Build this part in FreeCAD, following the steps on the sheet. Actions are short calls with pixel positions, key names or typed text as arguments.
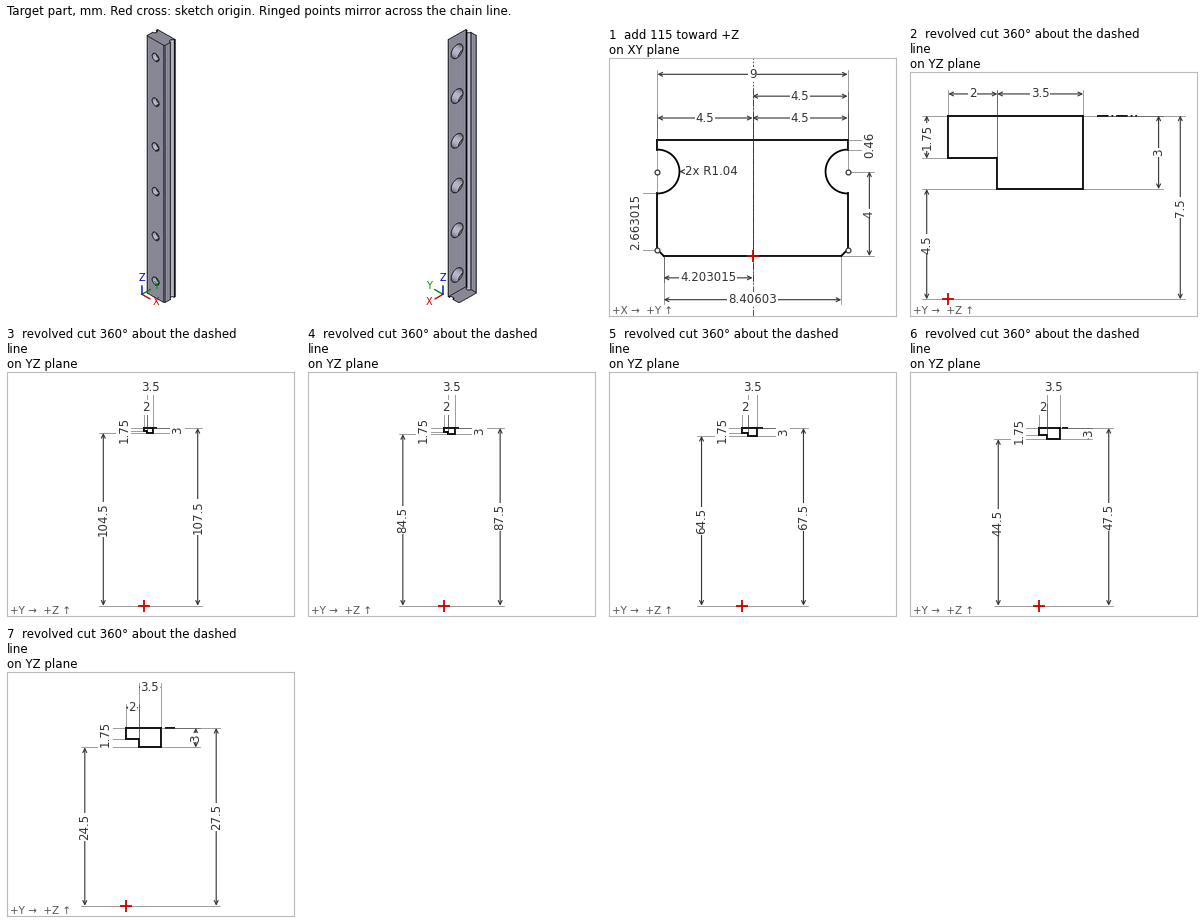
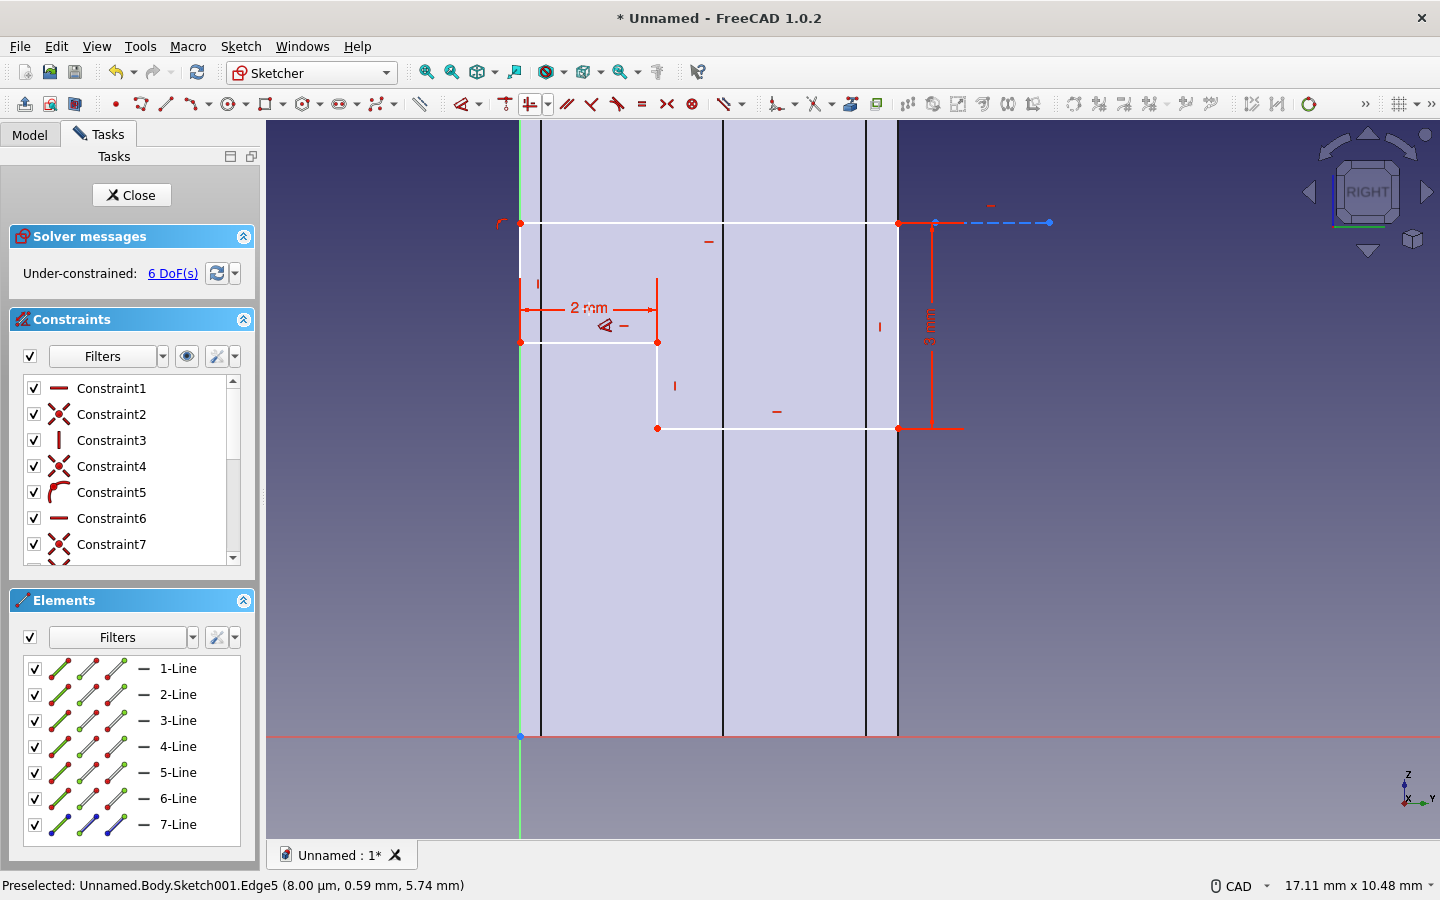
click(730, 429)
click(778, 395)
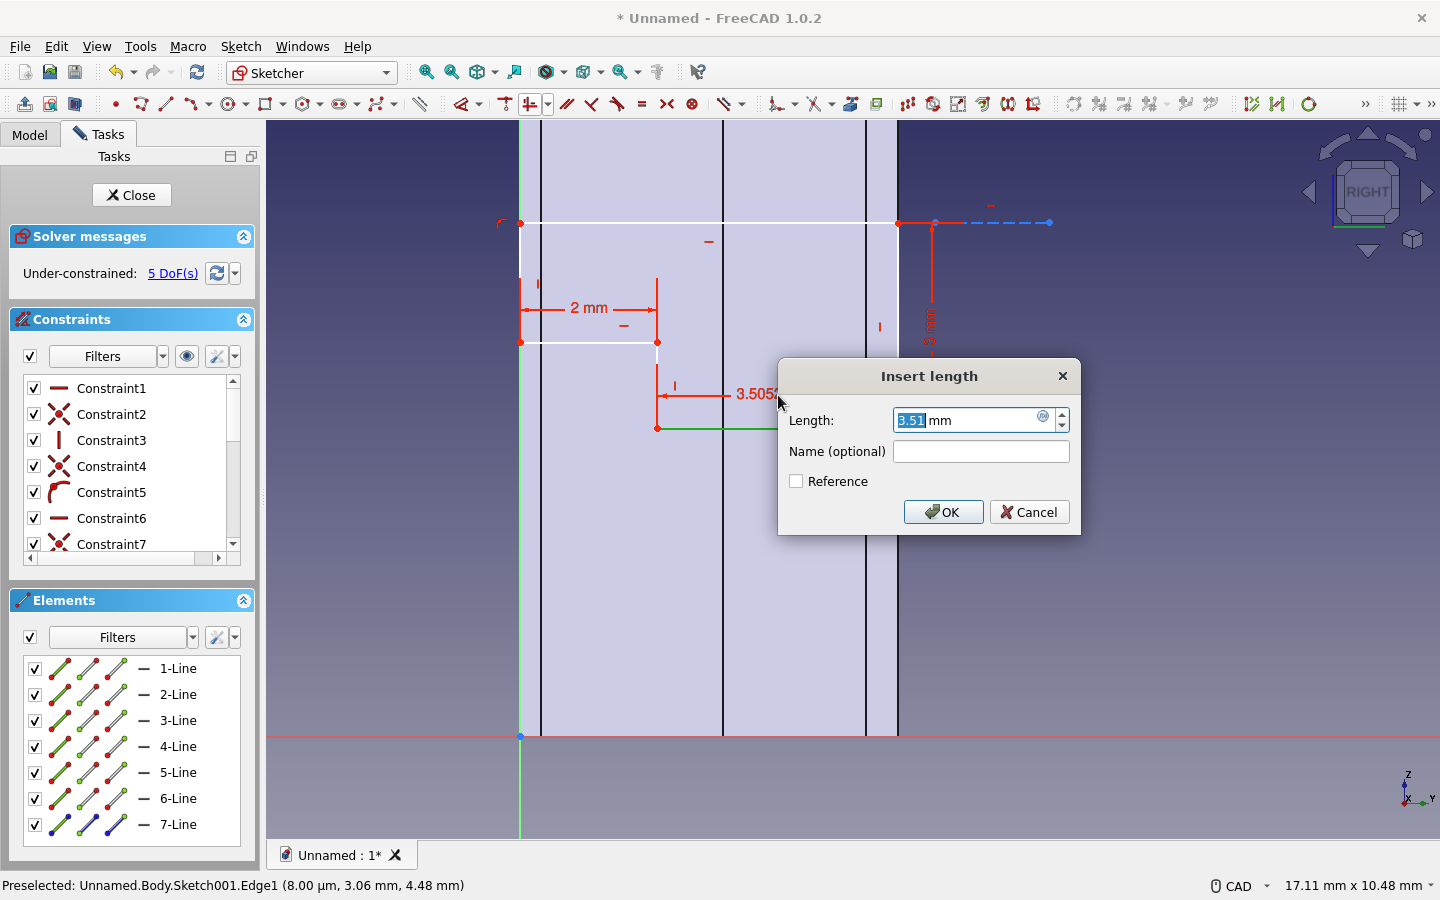
text(3.5)
key(Return)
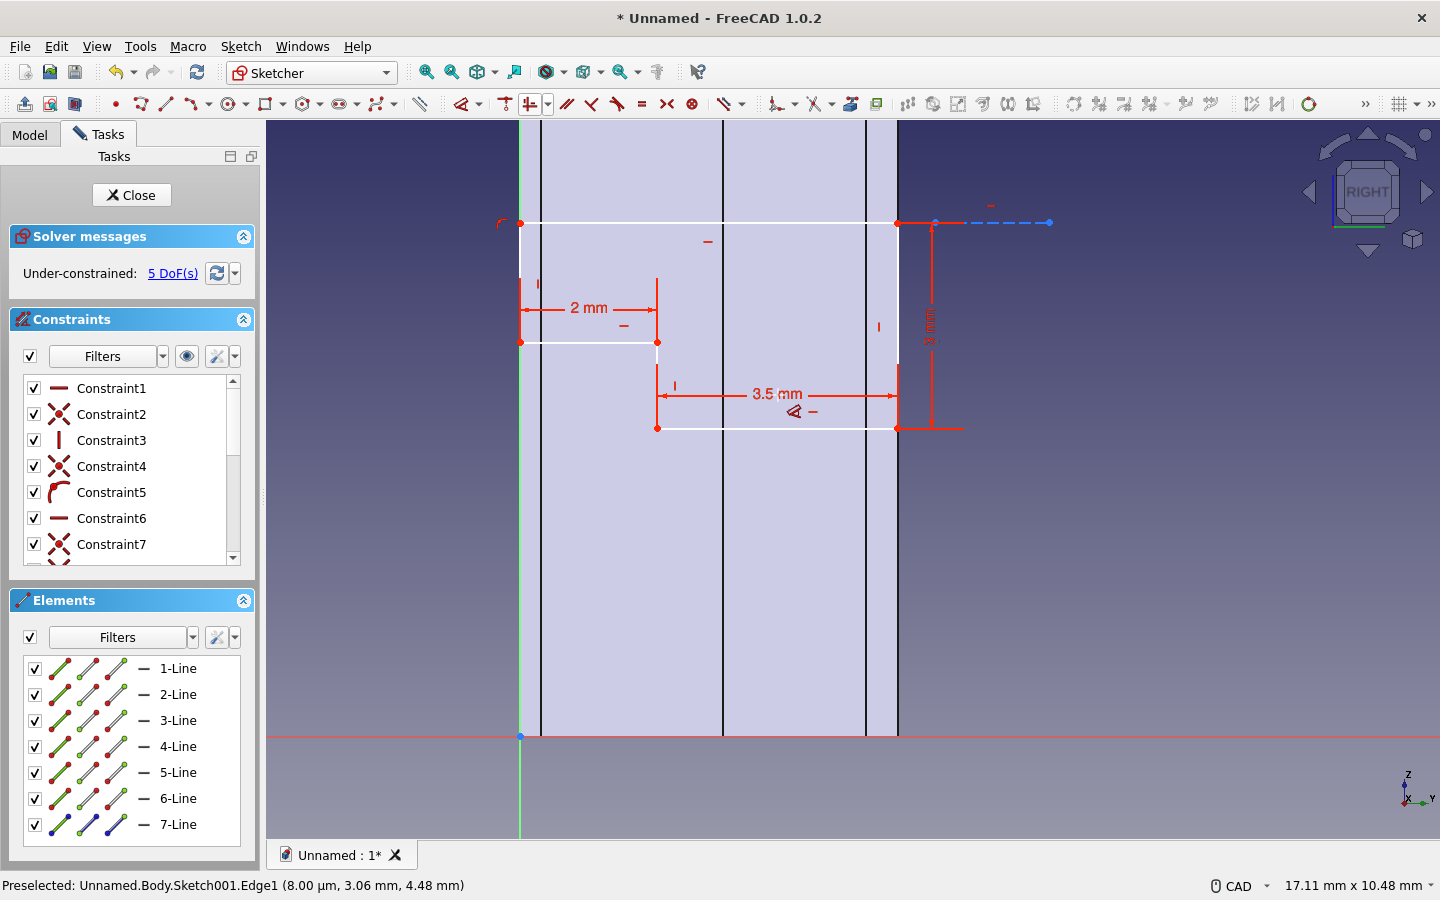
click(520, 259)
click(486, 283)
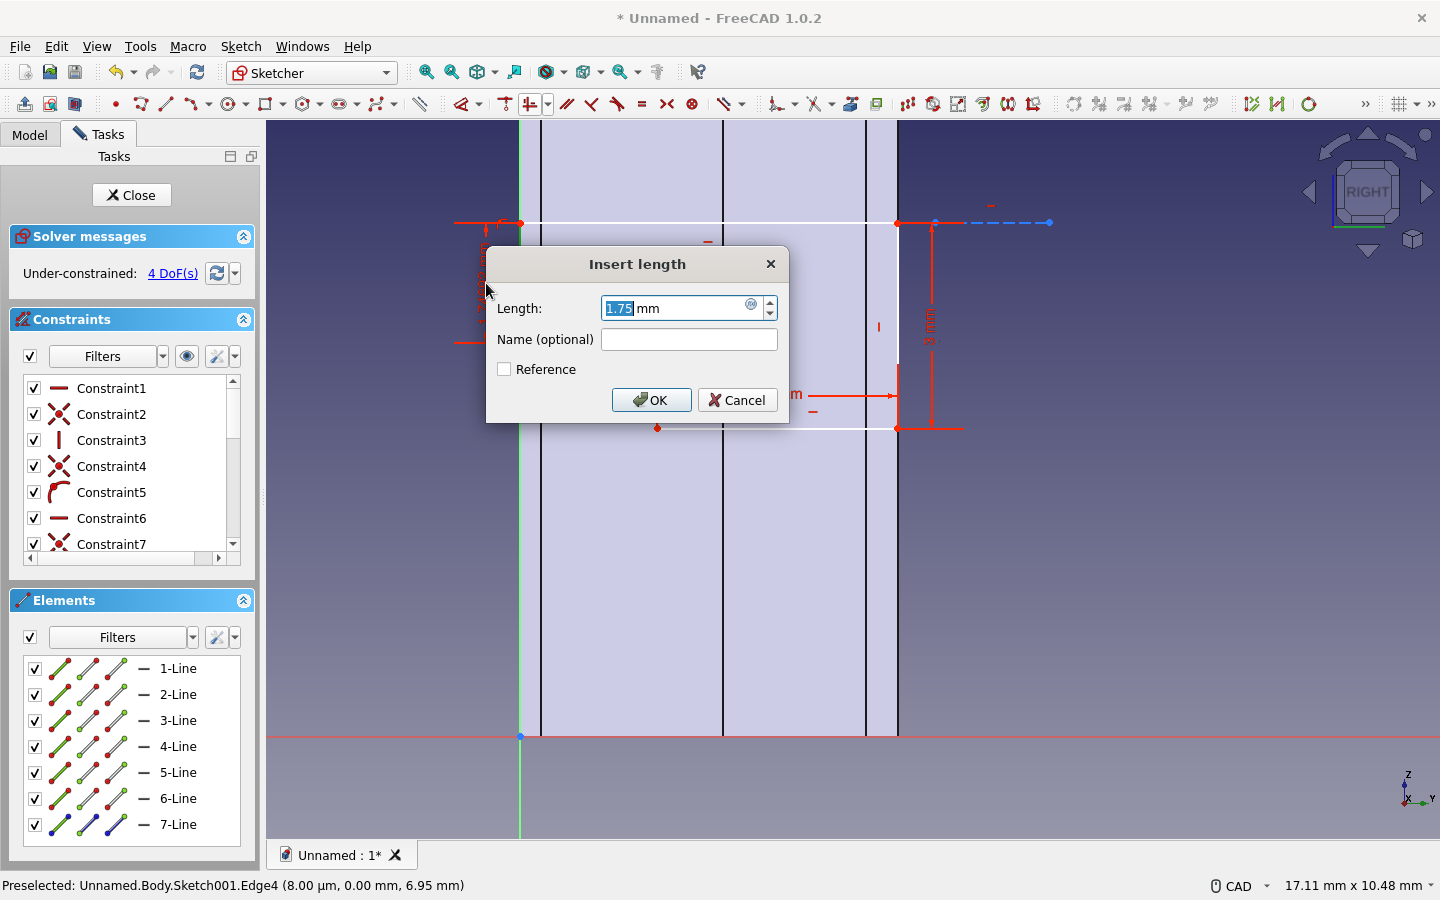
text(1.75)
key(Return)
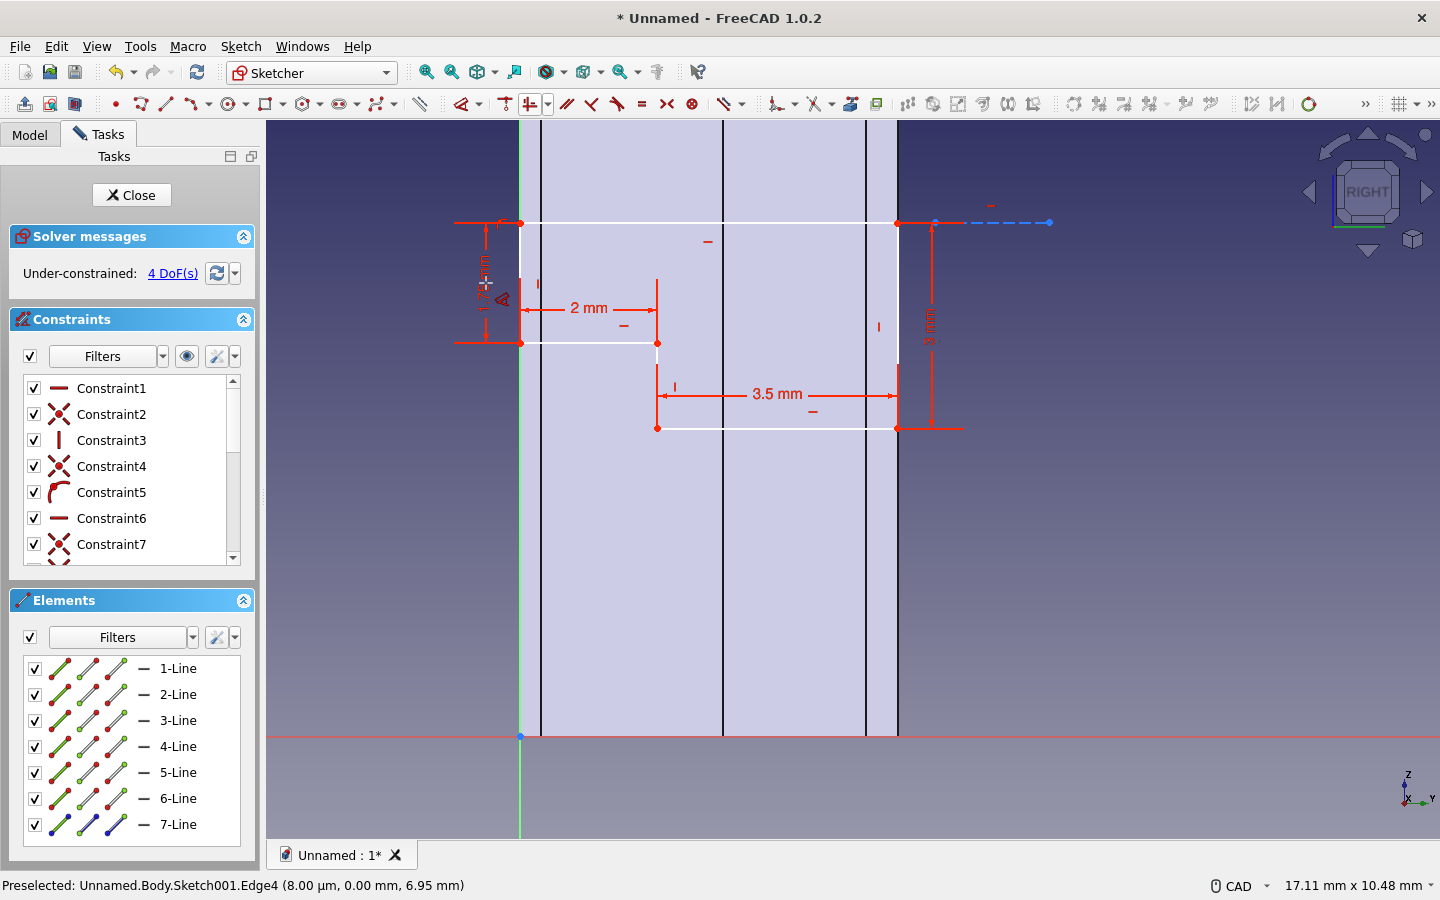
click(657, 429)
click(486, 583)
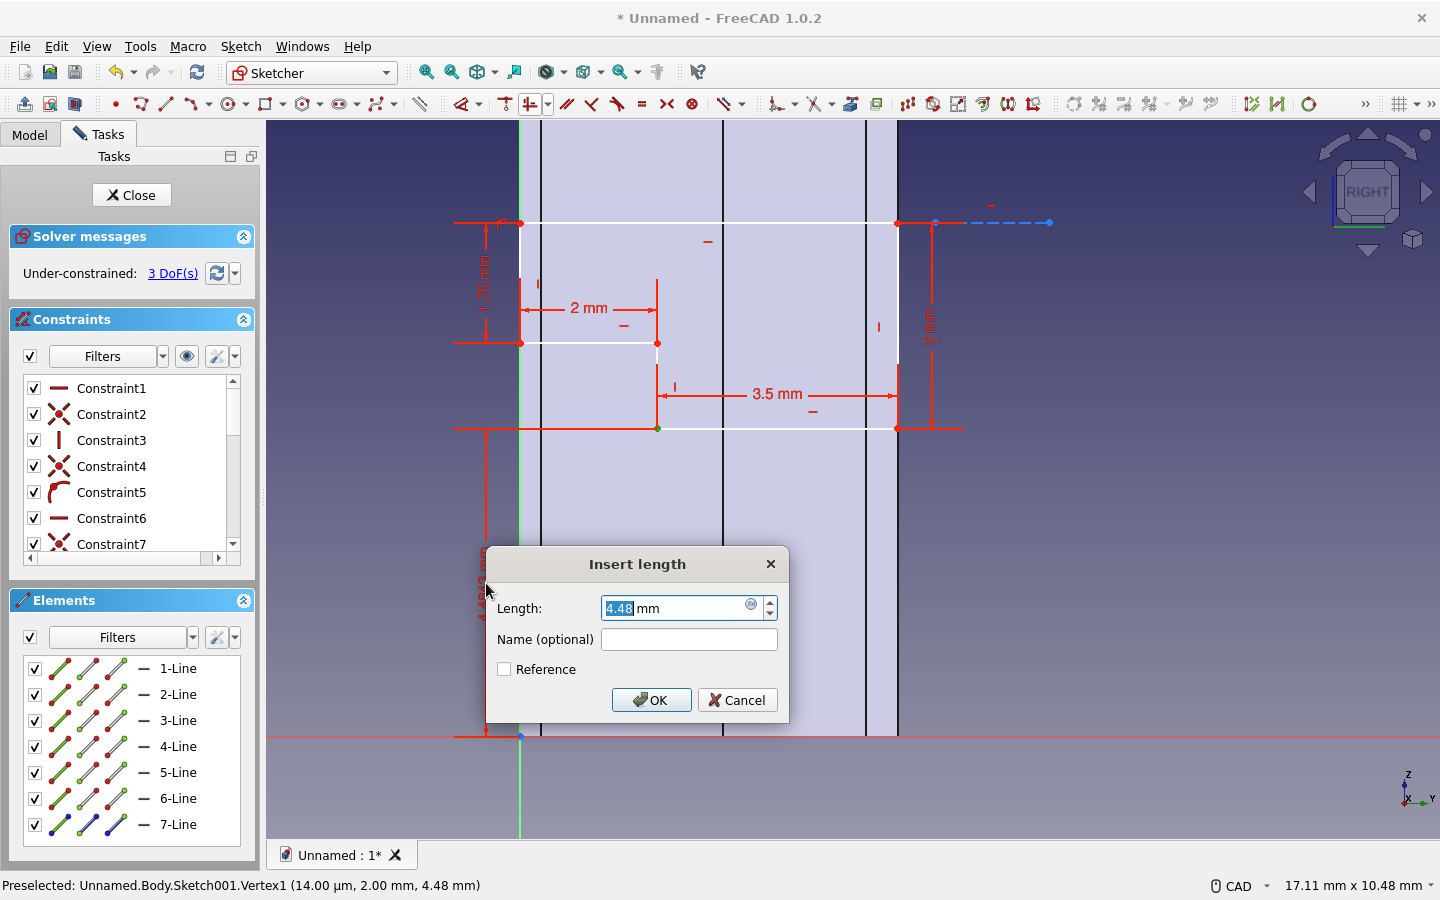
text(4.5)
key(Return)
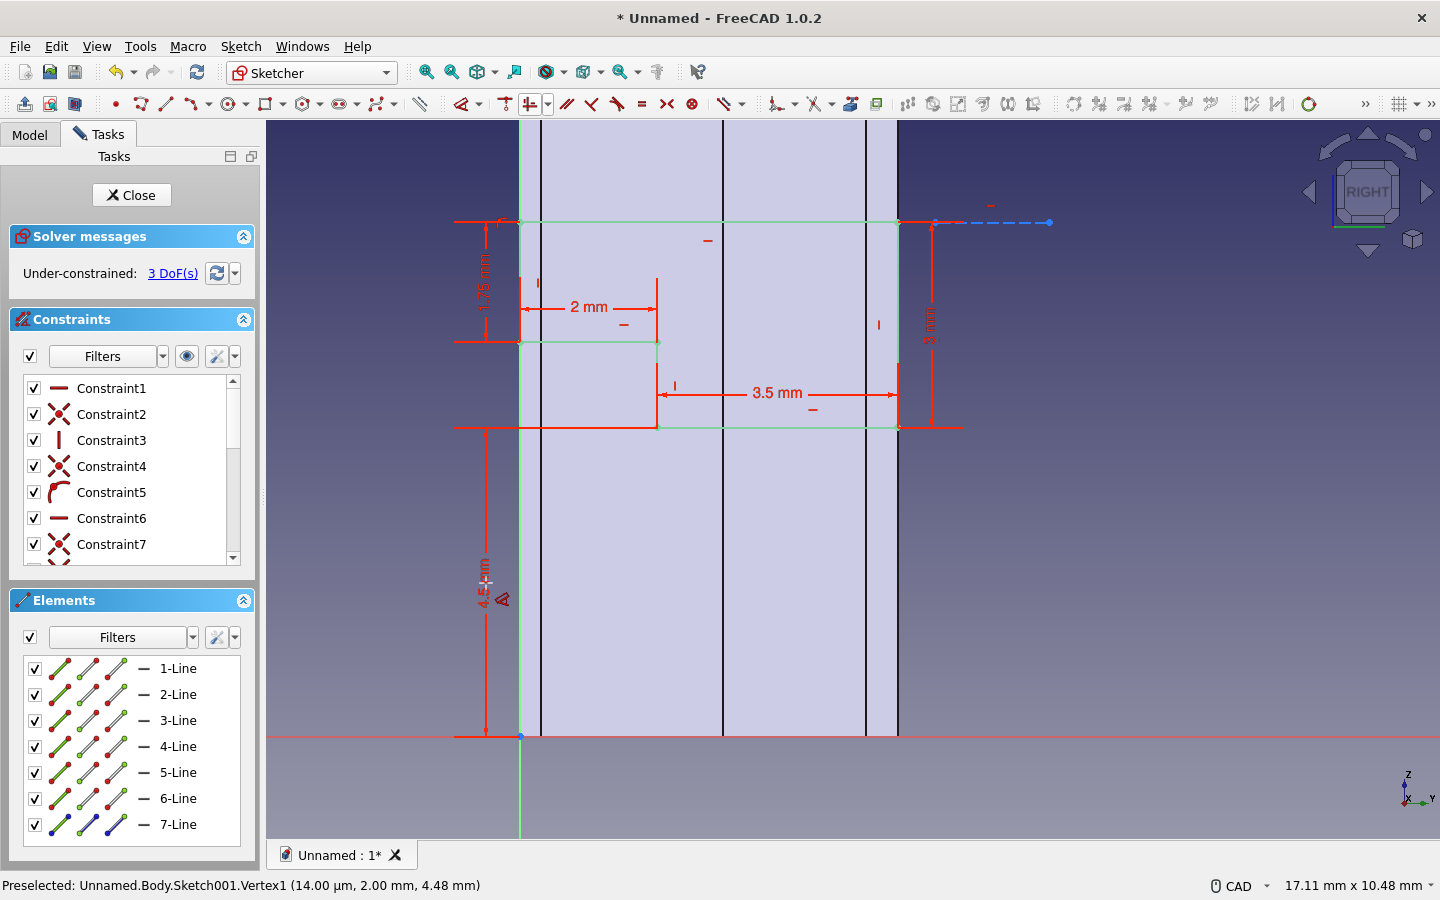
click(935, 223)
click(486, 480)